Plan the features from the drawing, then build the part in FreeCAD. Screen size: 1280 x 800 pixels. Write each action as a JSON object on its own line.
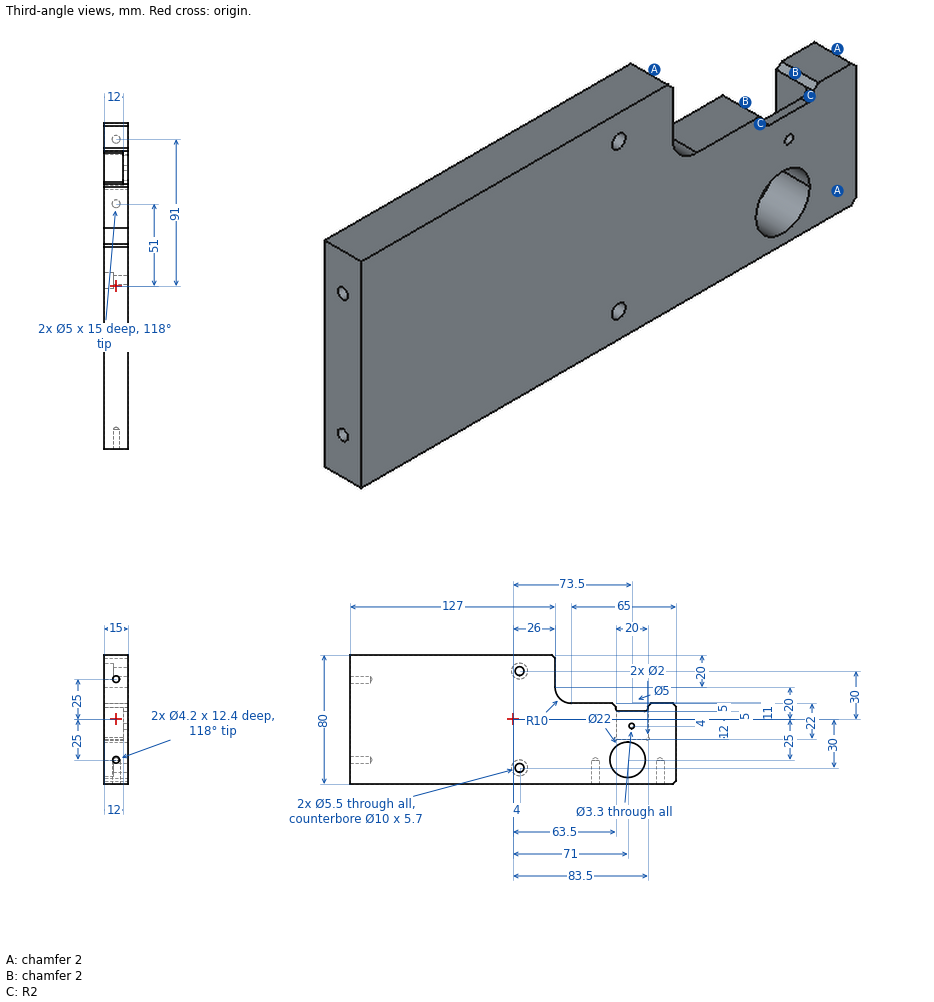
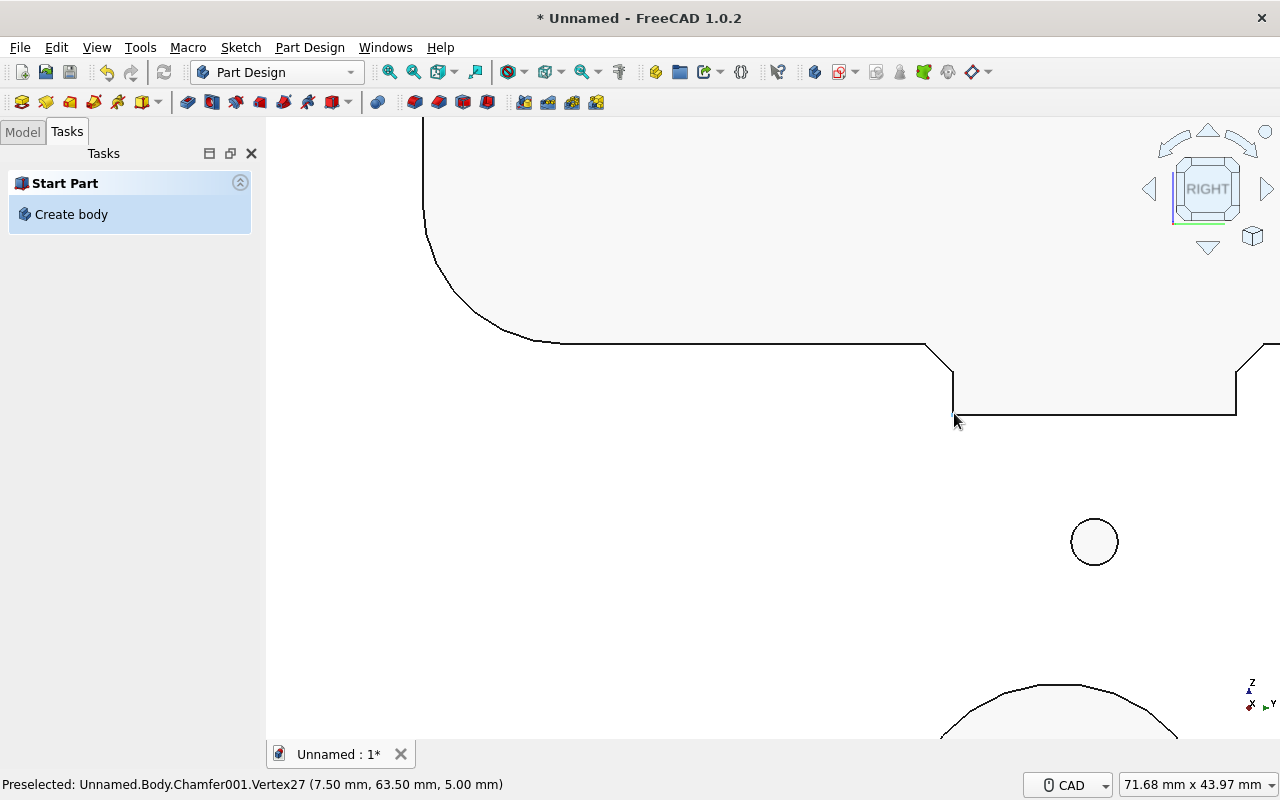
{"action": "left_click", "coordinate": [390, 72]}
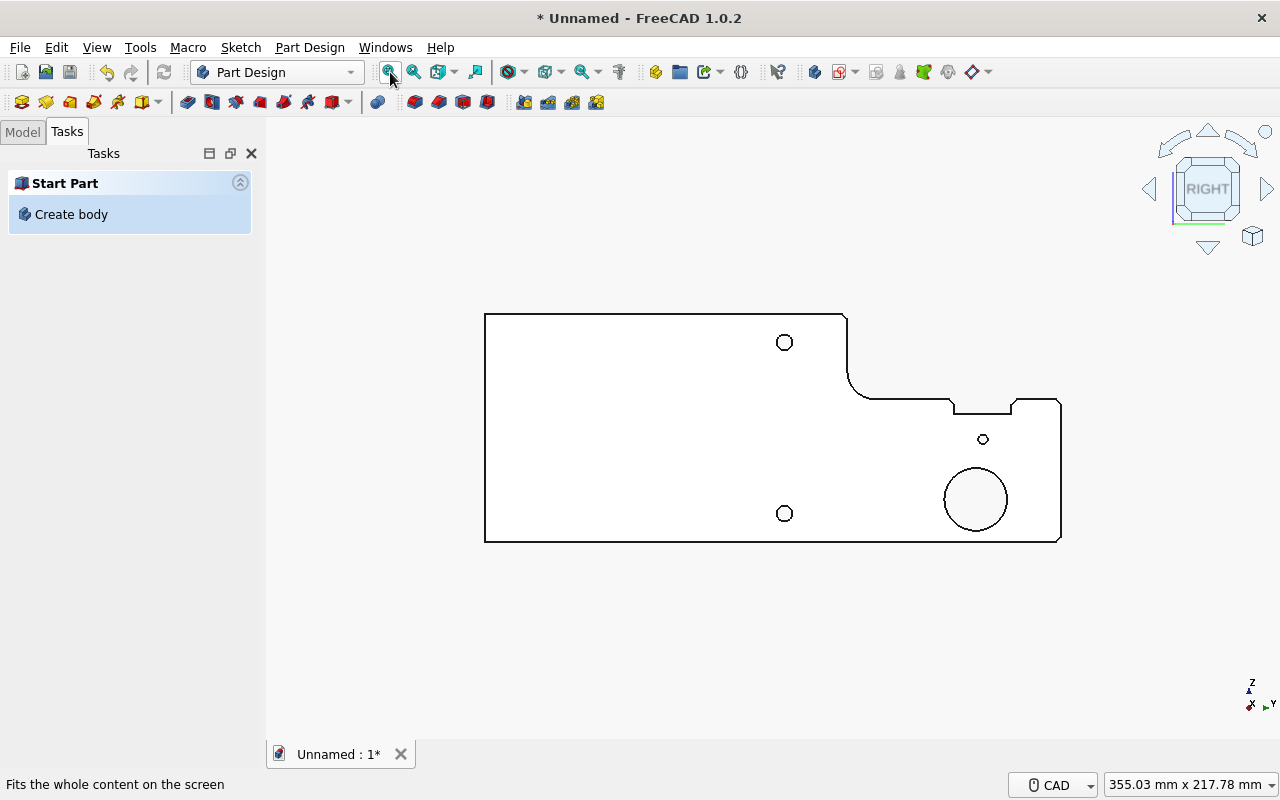
{"action": "key", "text": "5"}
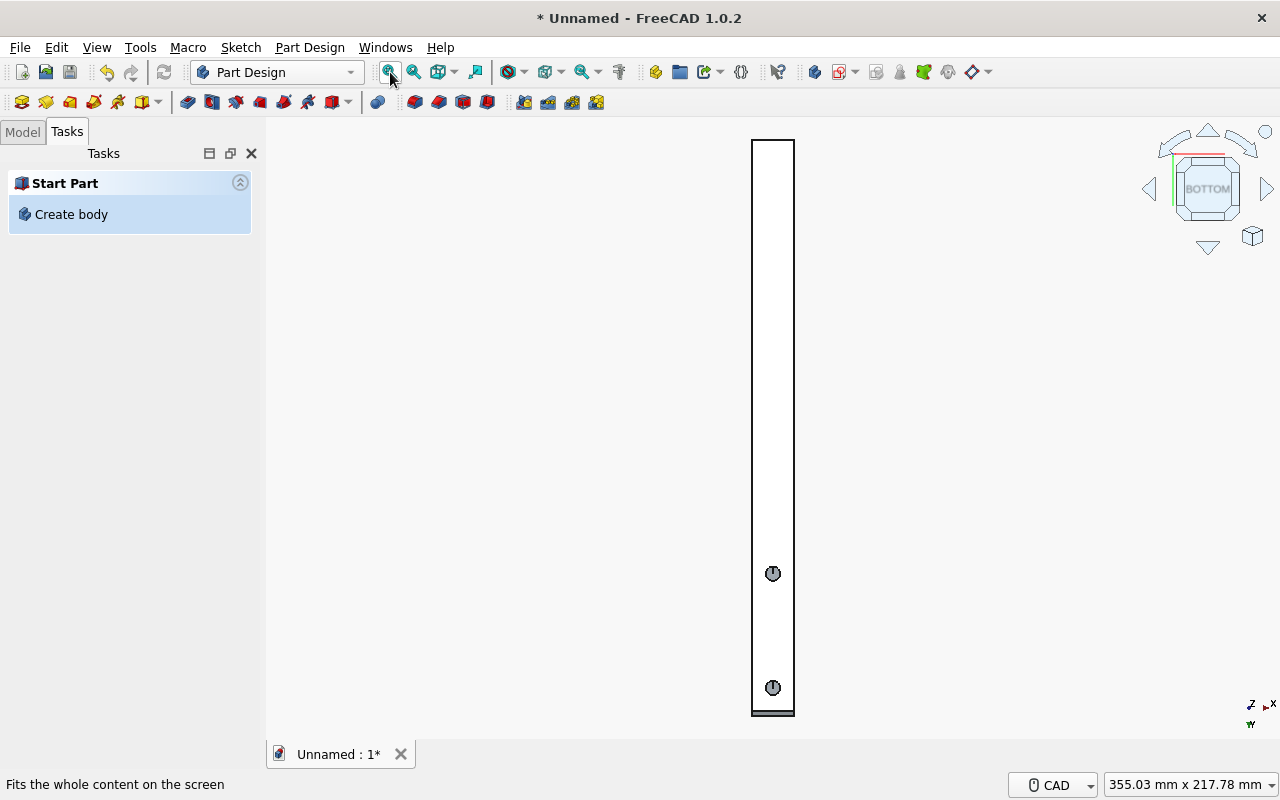
{"action": "scroll", "coordinate": [790, 608], "scroll_direction": "up", "scroll_amount": 8}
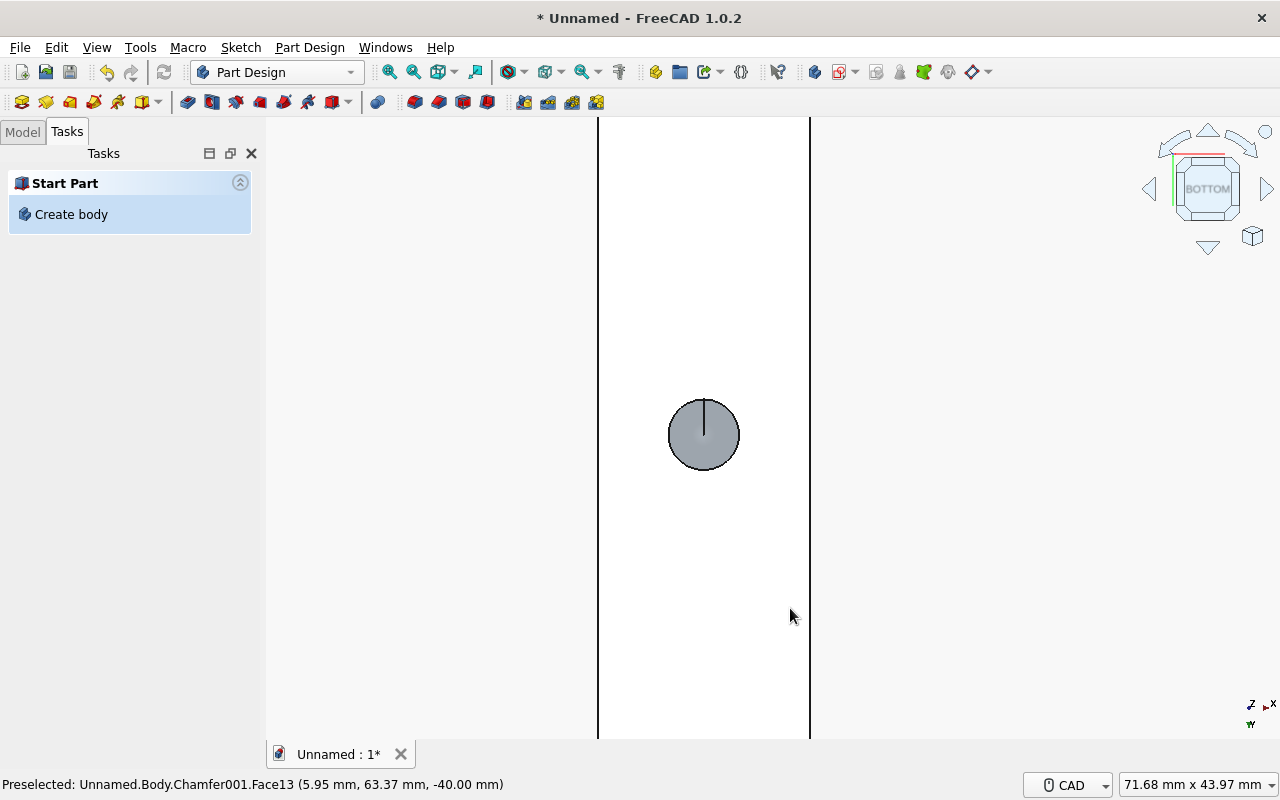
{"action": "left_click", "coordinate": [390, 72]}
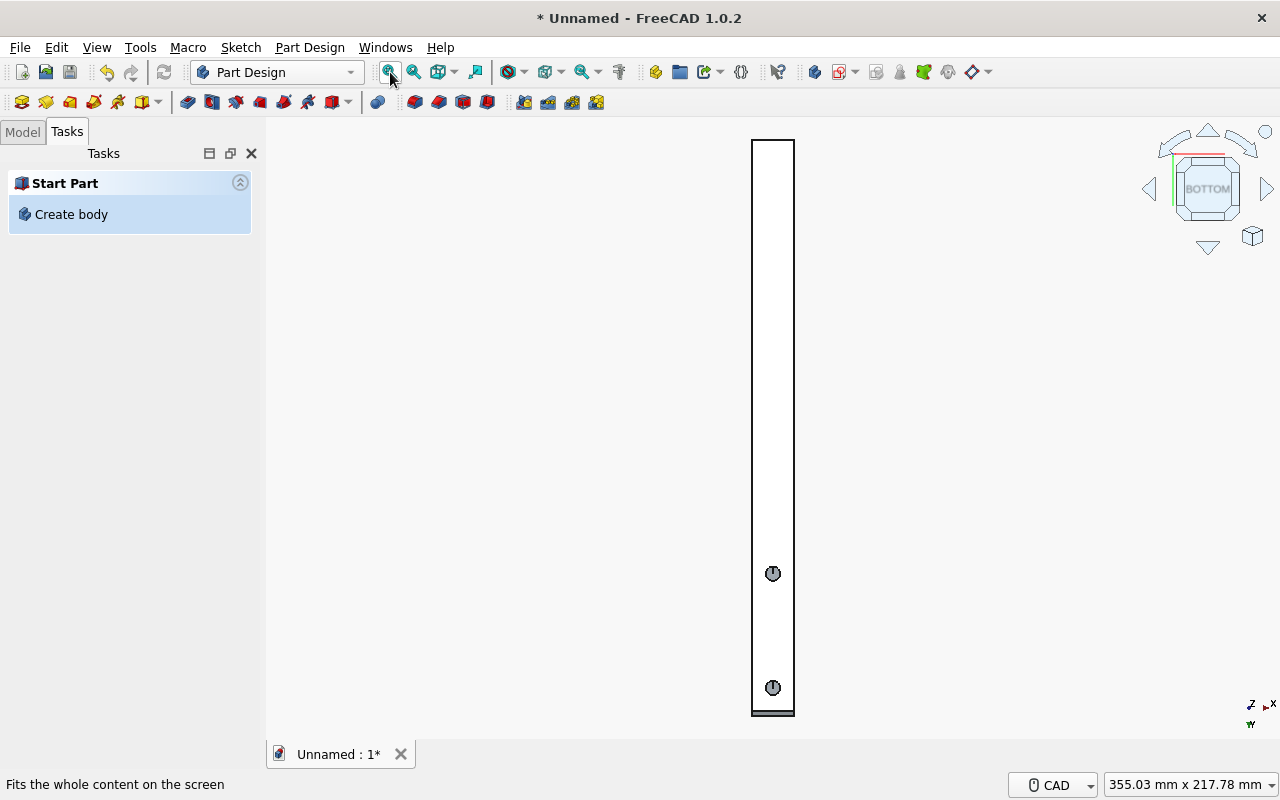
{"action": "key", "text": "4"}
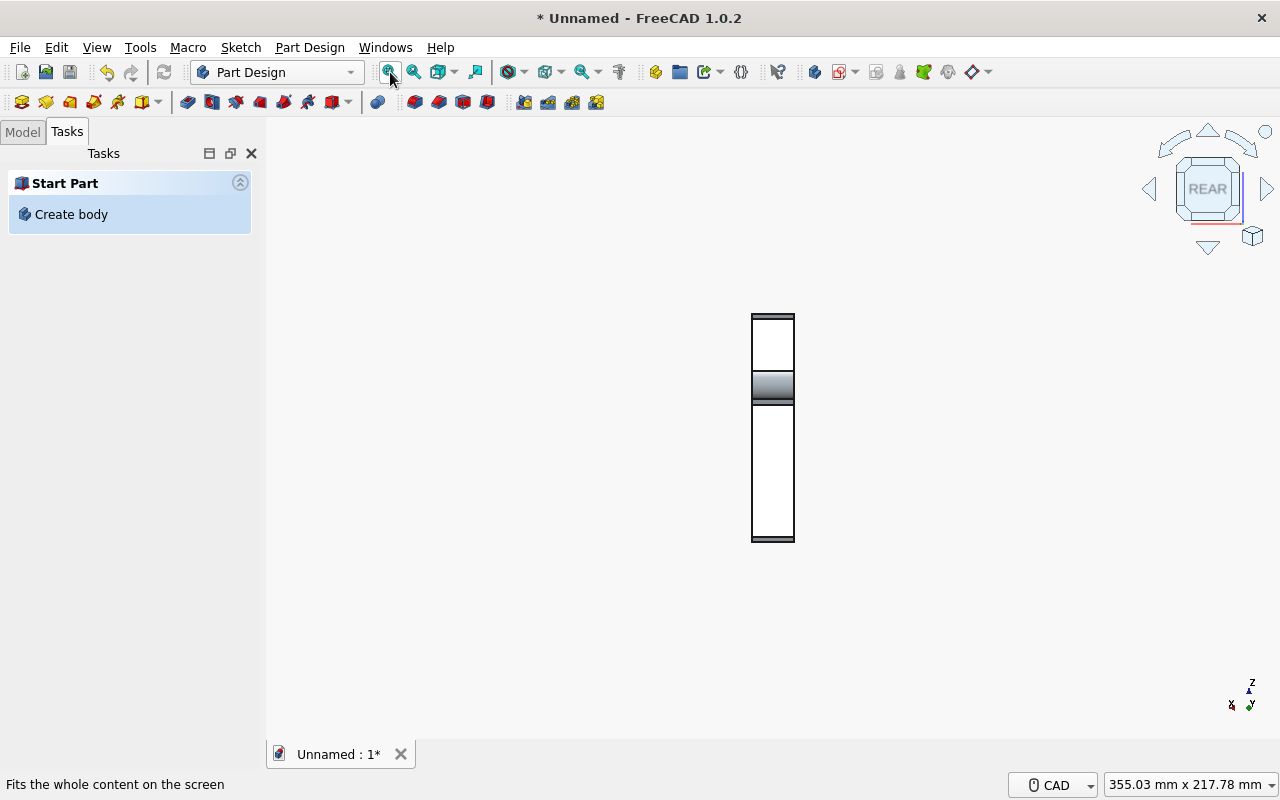
{"action": "left_click", "coordinate": [390, 72]}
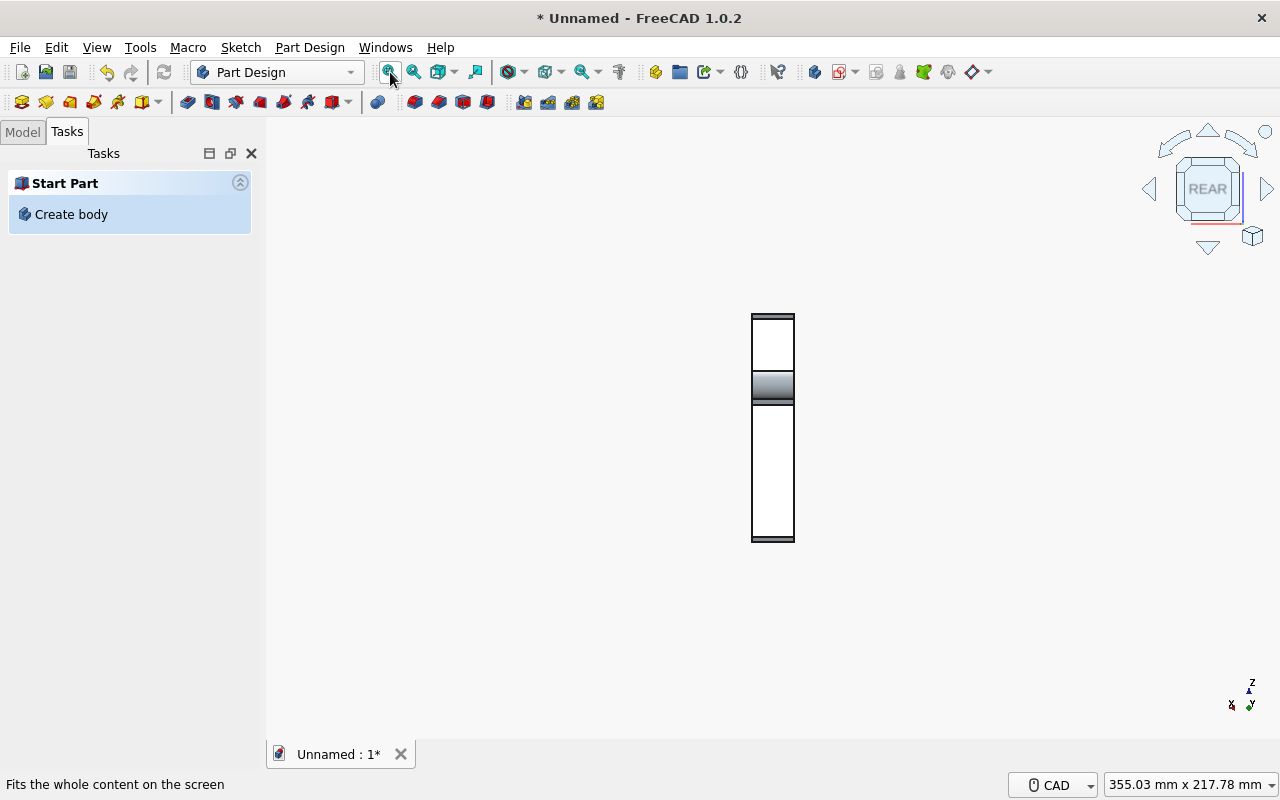
{"action": "scroll", "coordinate": [756, 413], "scroll_direction": "up", "scroll_amount": 8}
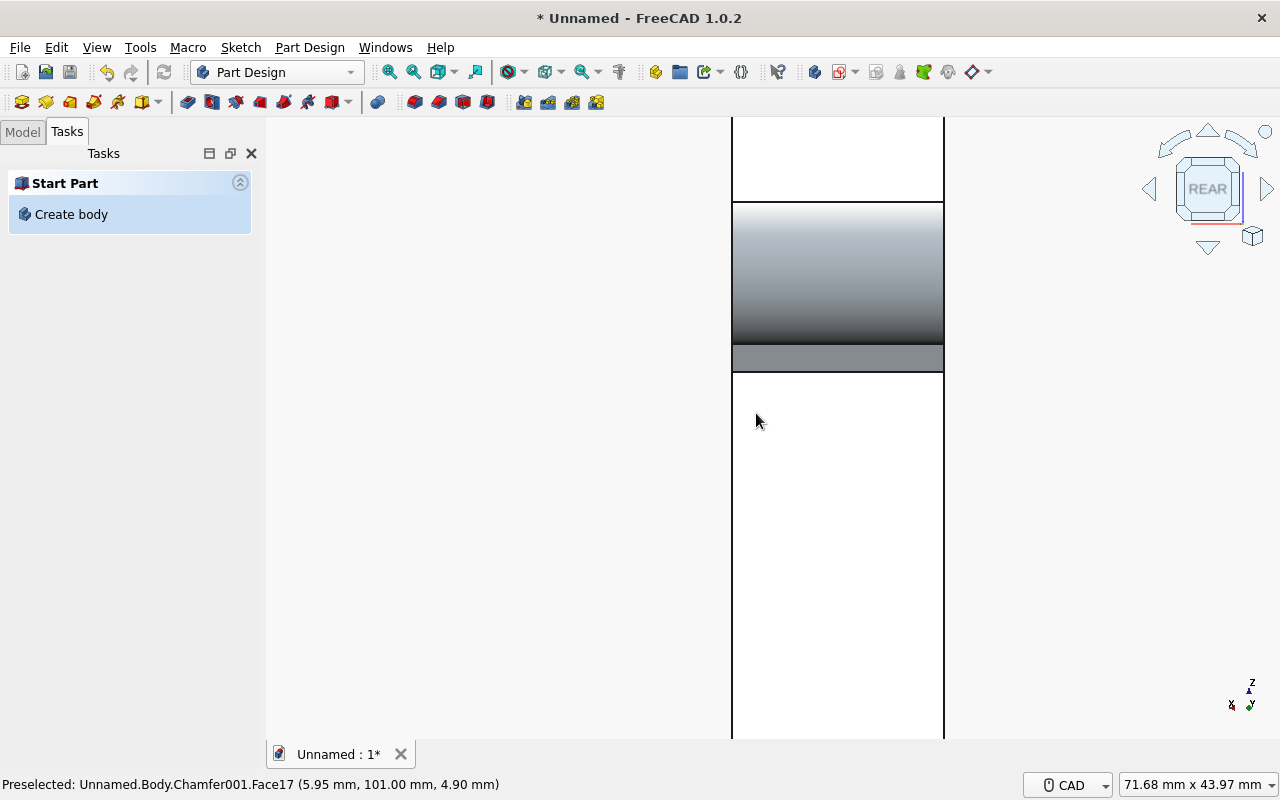
{"action": "left_click", "coordinate": [390, 72]}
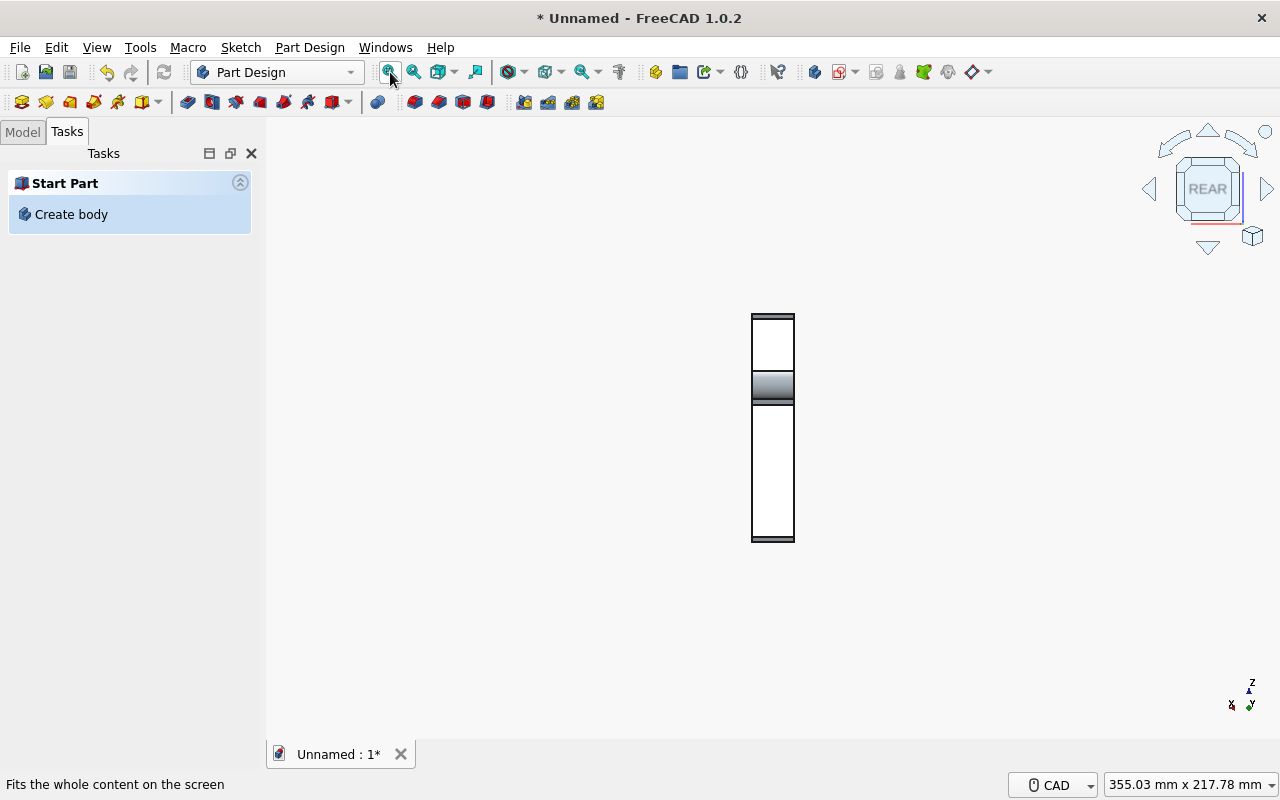
{"action": "key", "text": "6"}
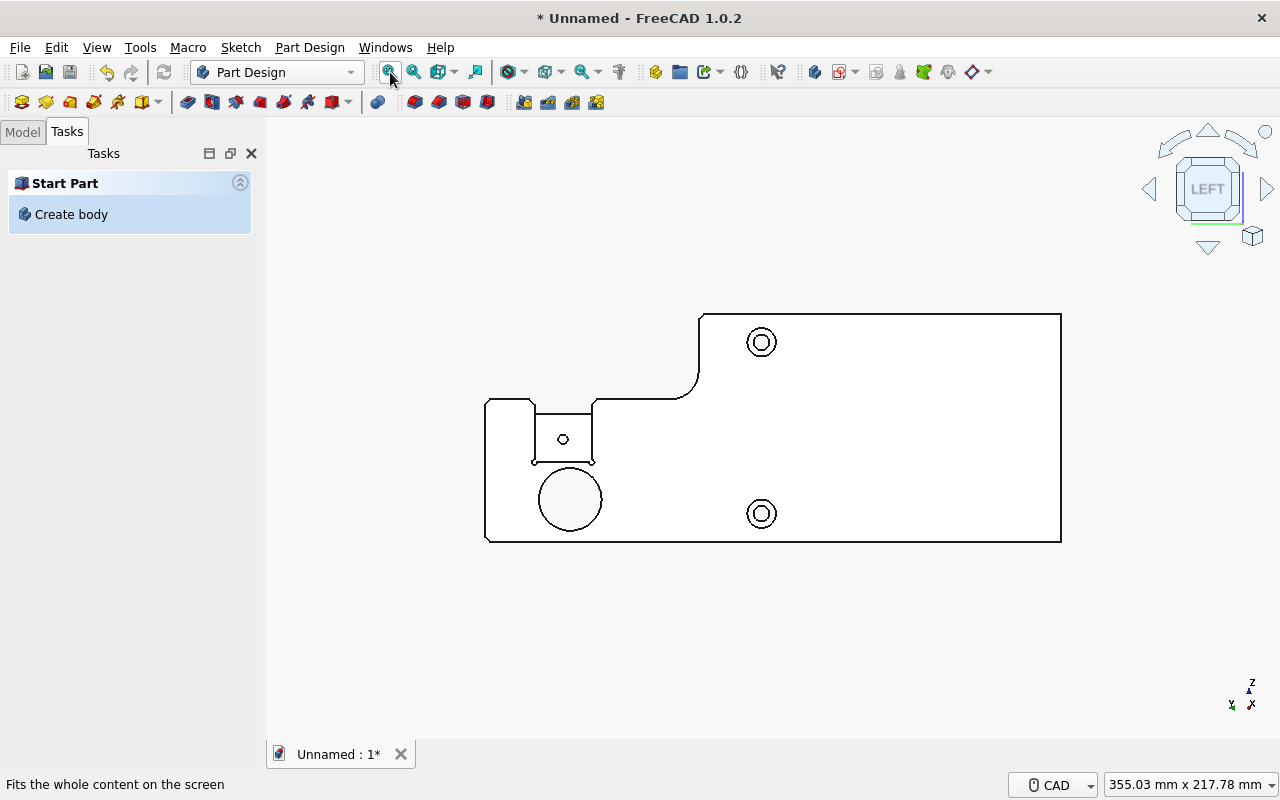
{"action": "scroll", "coordinate": [592, 413], "scroll_direction": "up", "scroll_amount": 8}